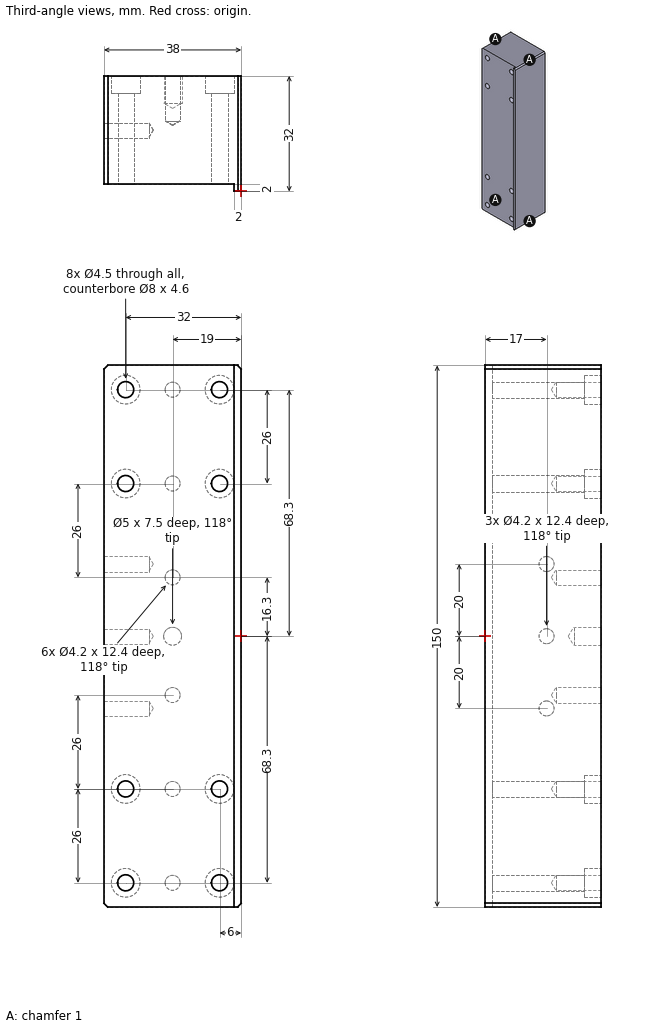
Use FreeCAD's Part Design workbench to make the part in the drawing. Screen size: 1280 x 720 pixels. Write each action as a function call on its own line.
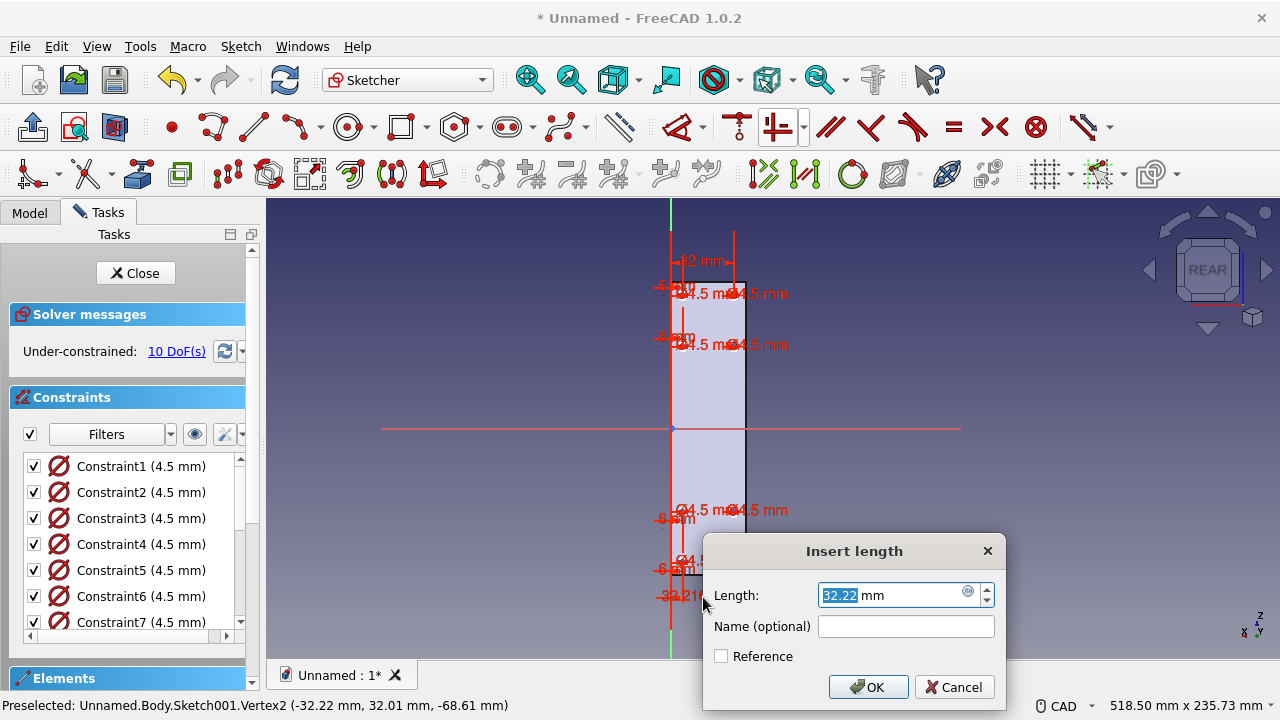
text(32)
key(Return)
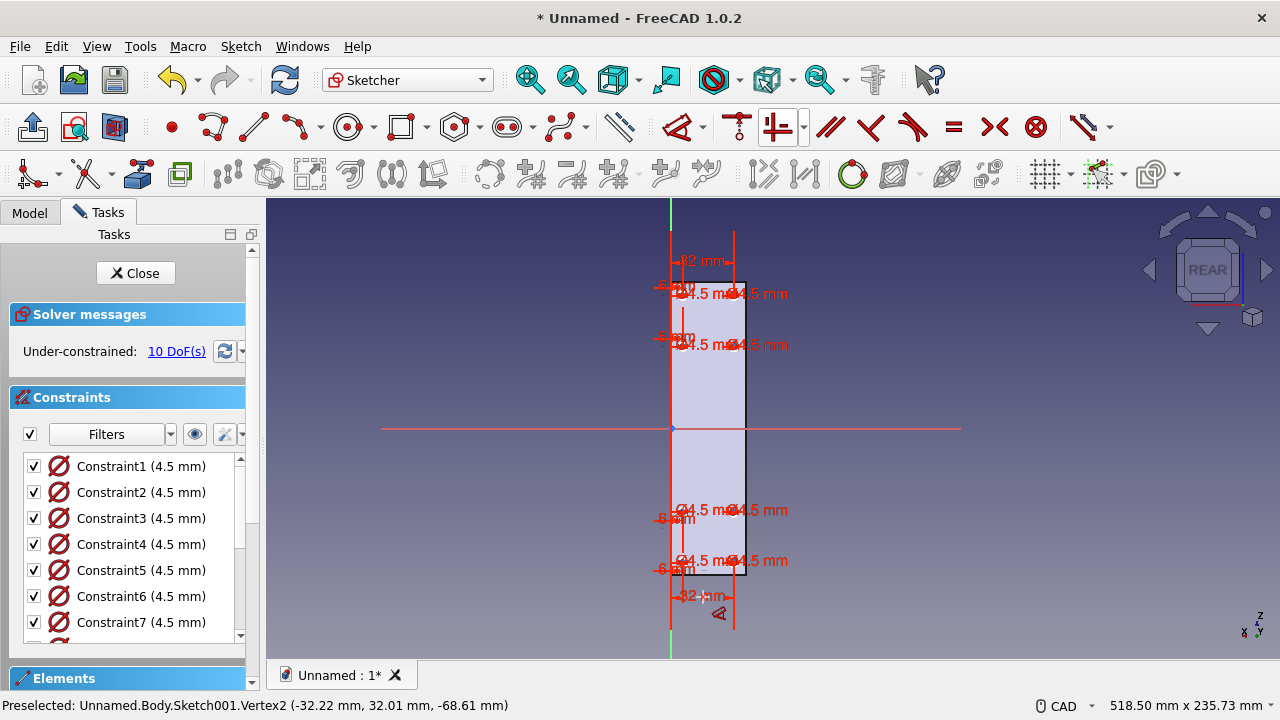
click(734, 512)
click(702, 546)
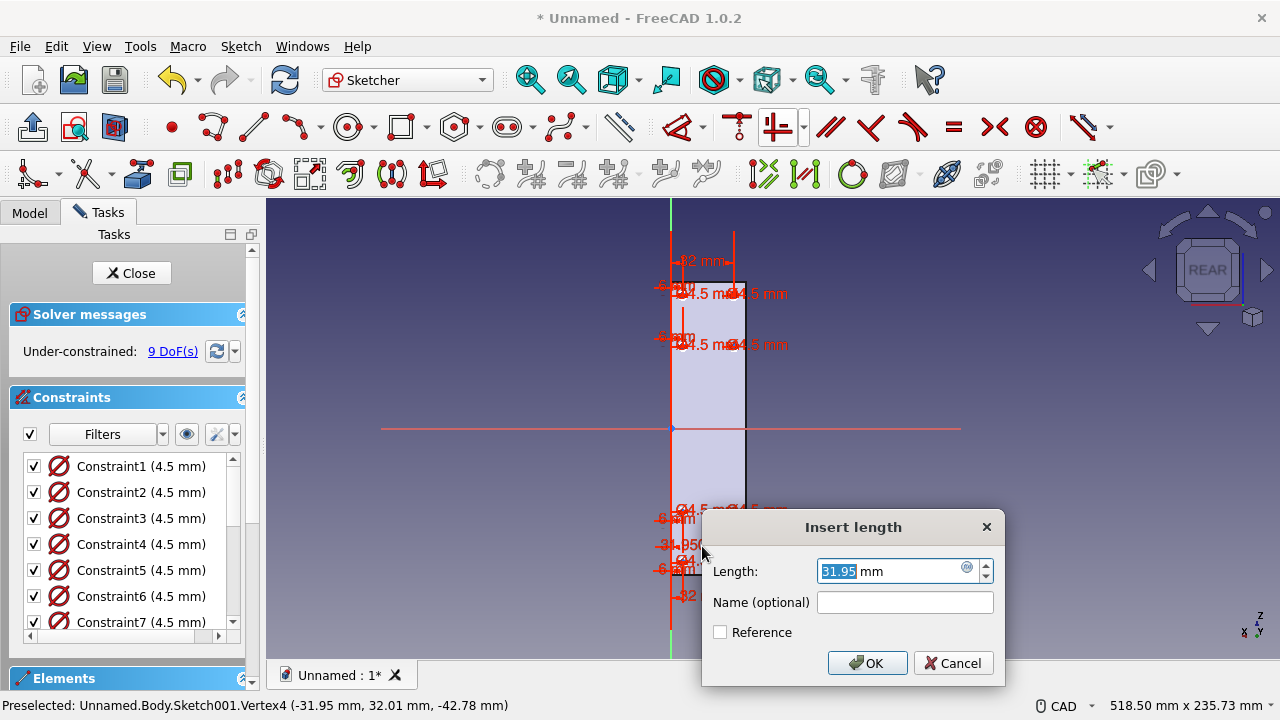
text(32)
key(Return)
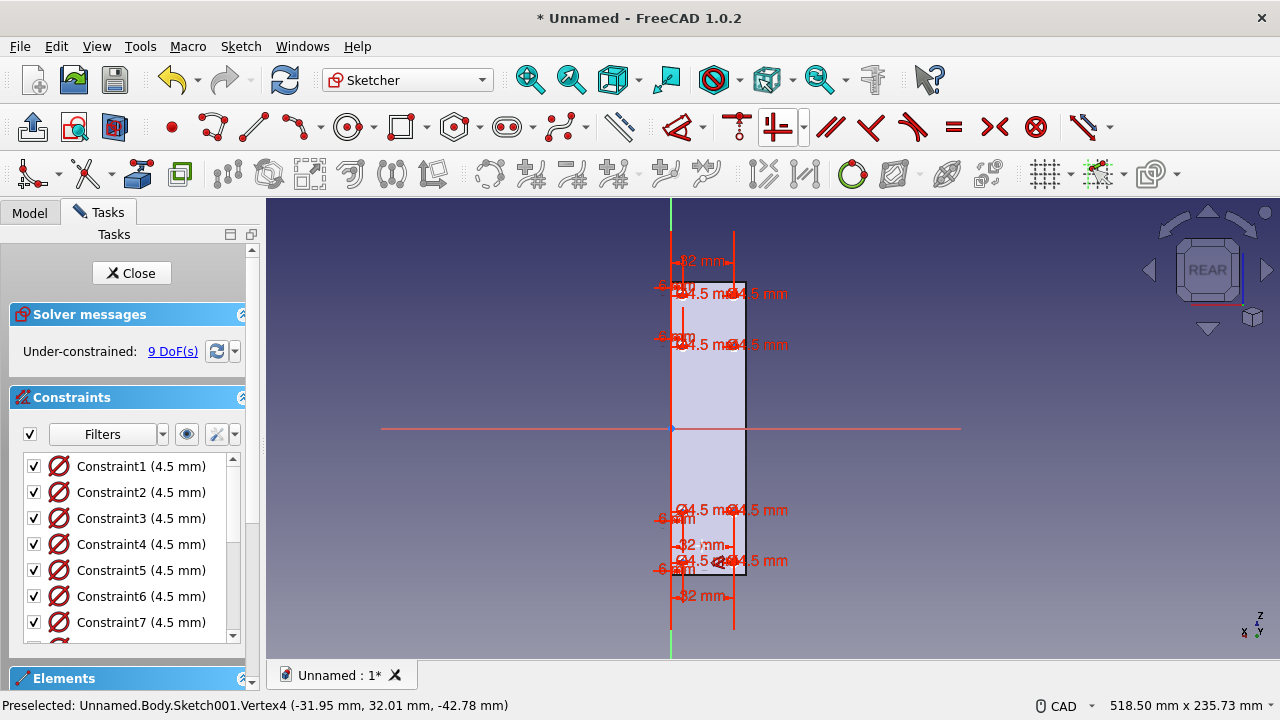
click(734, 347)
click(703, 313)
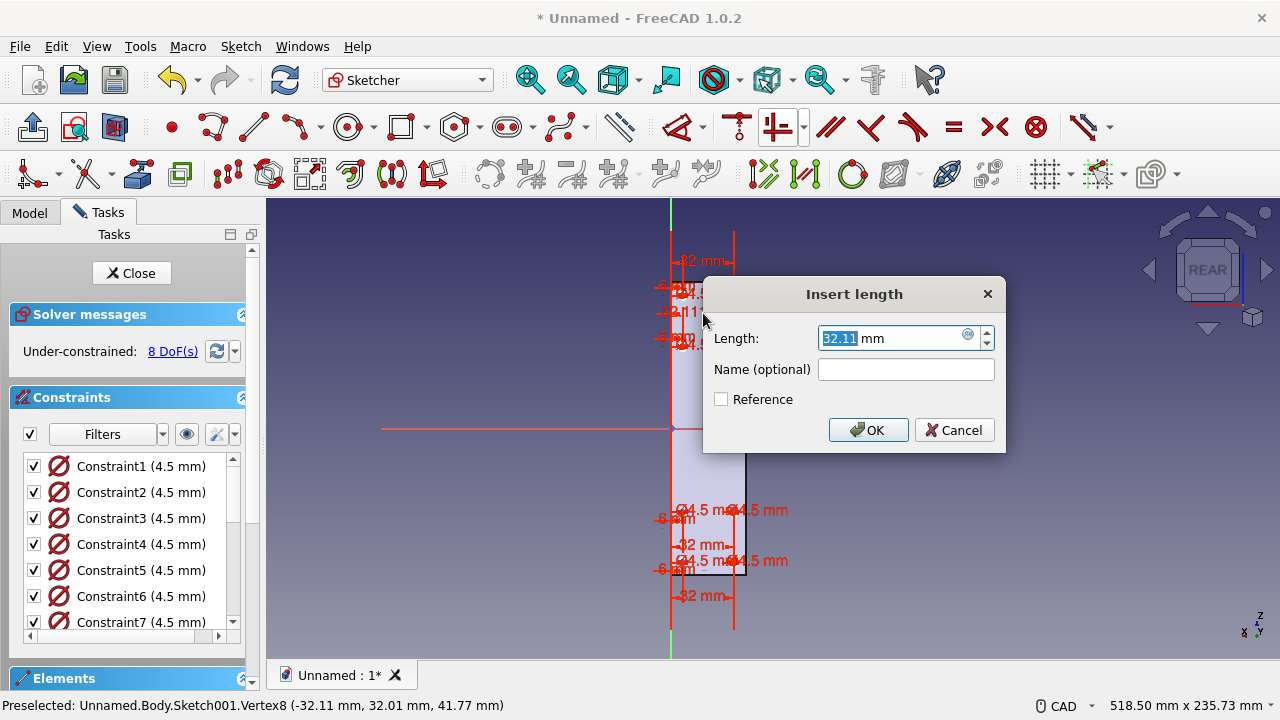
text(32)
key(Return)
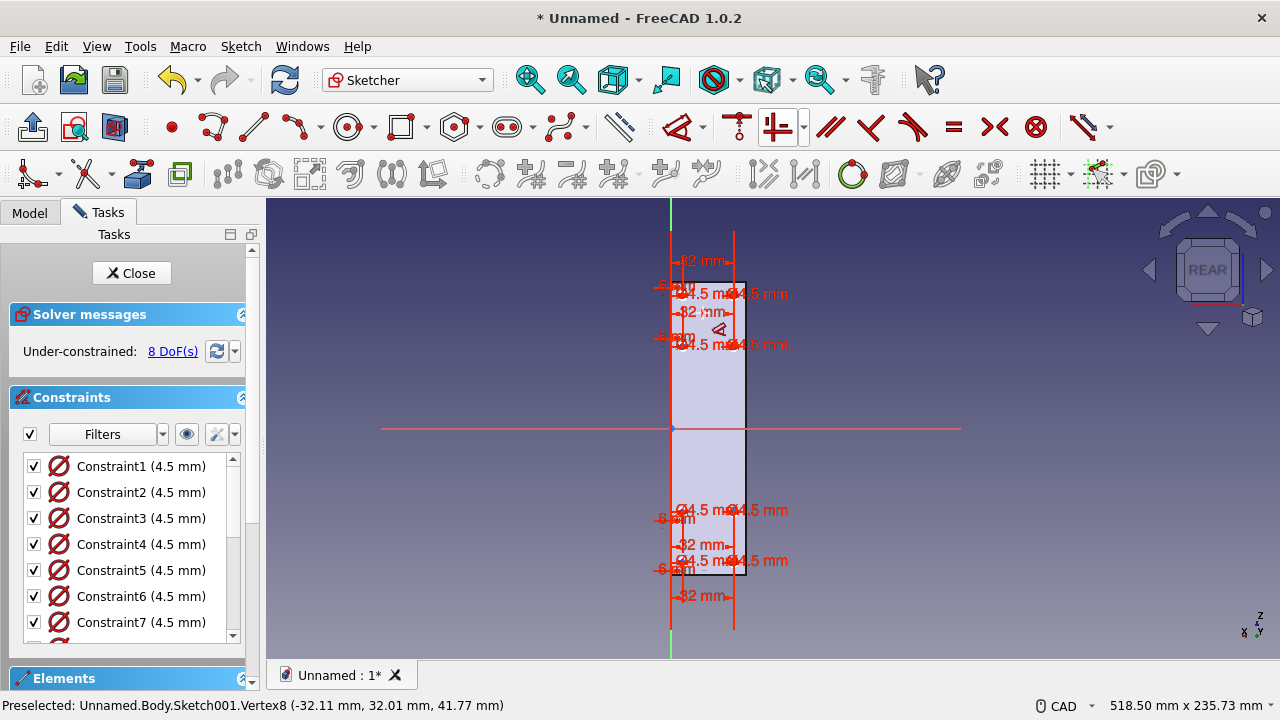
click(734, 563)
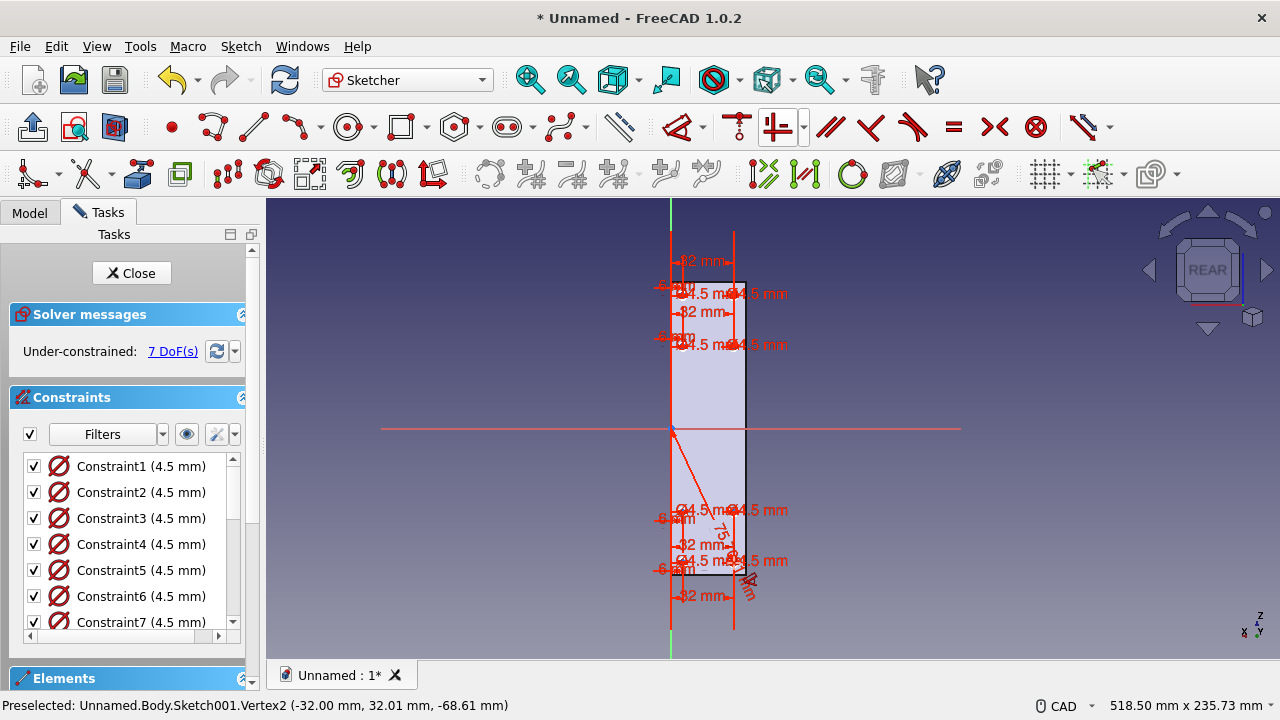
click(683, 512)
click(768, 526)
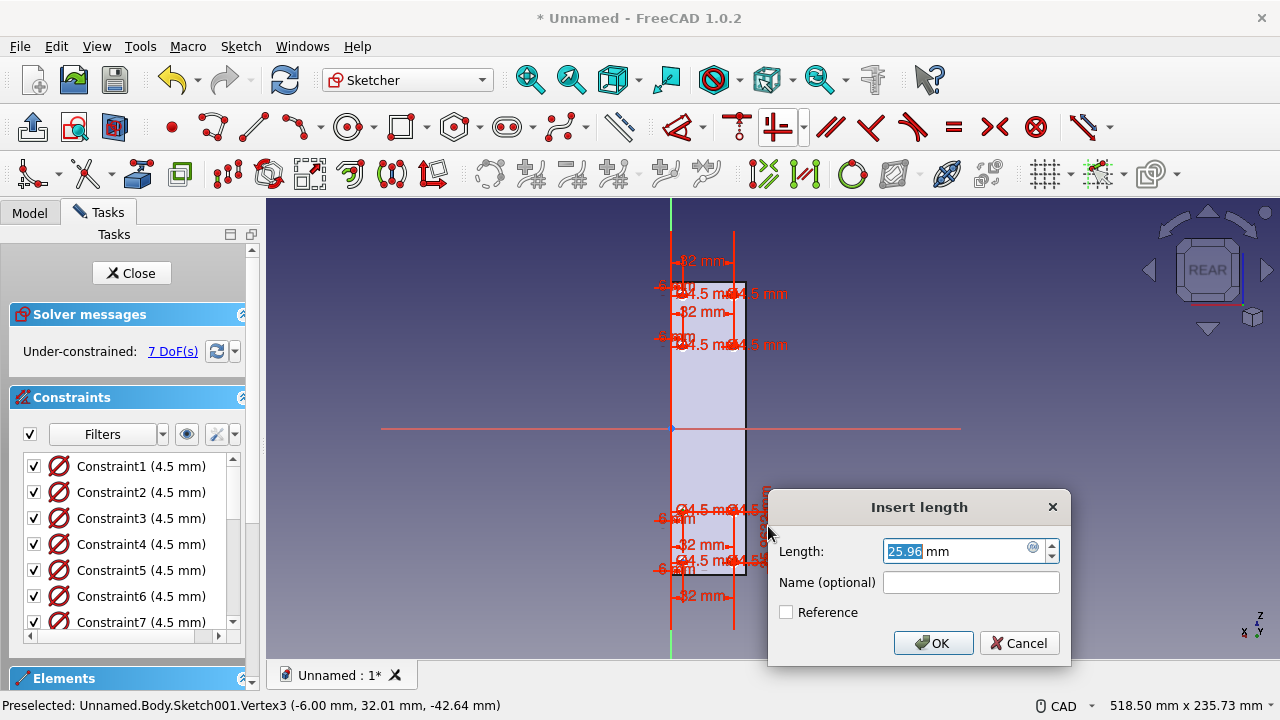
text(26)
key(Return)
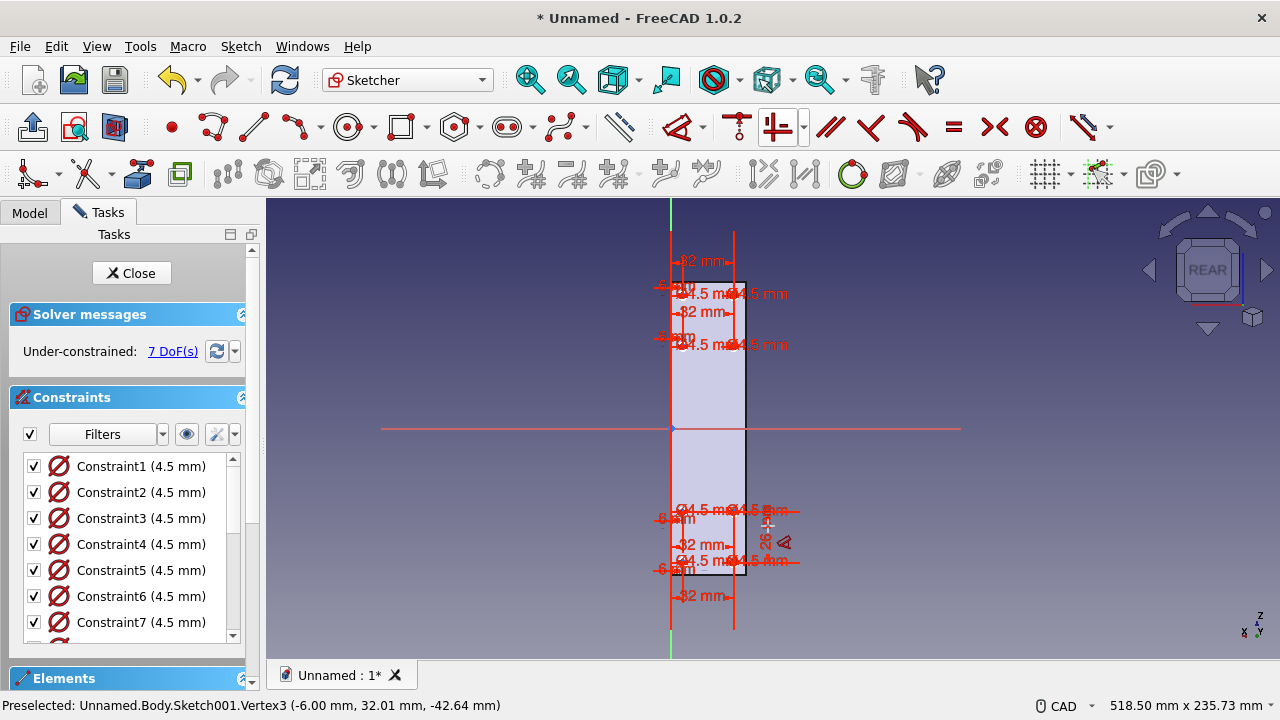
click(734, 563)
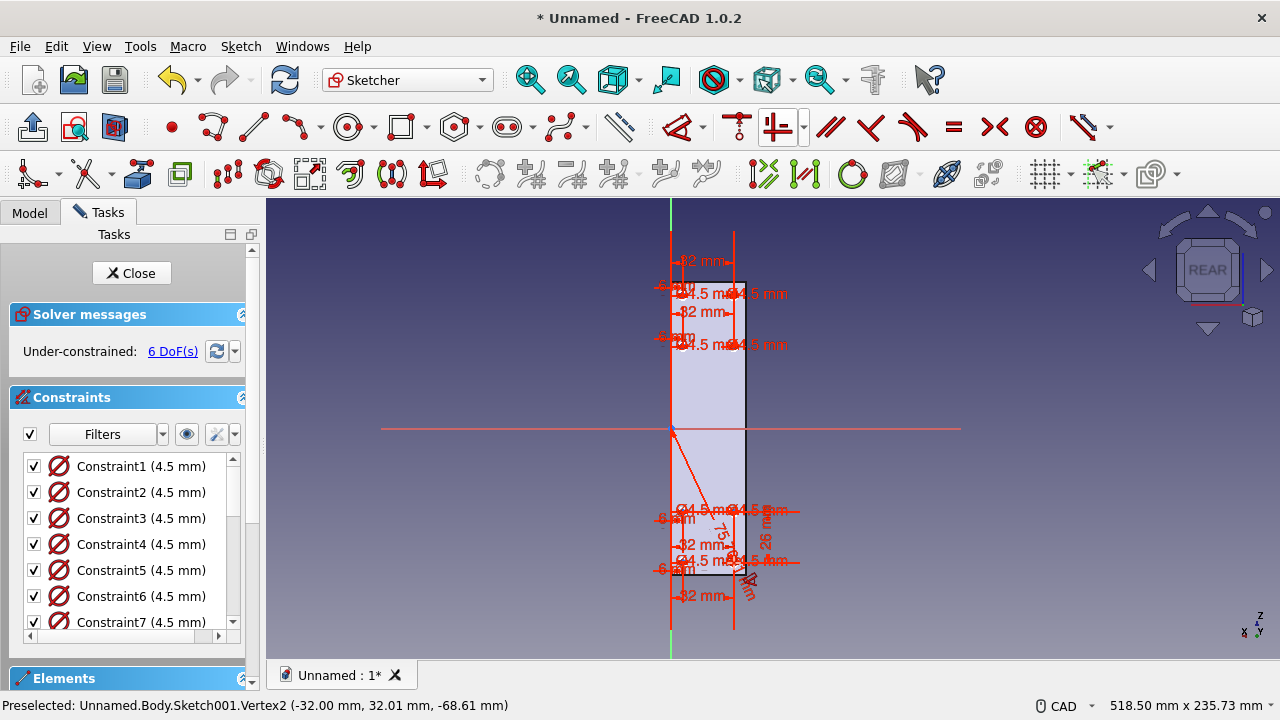
click(734, 512)
click(792, 549)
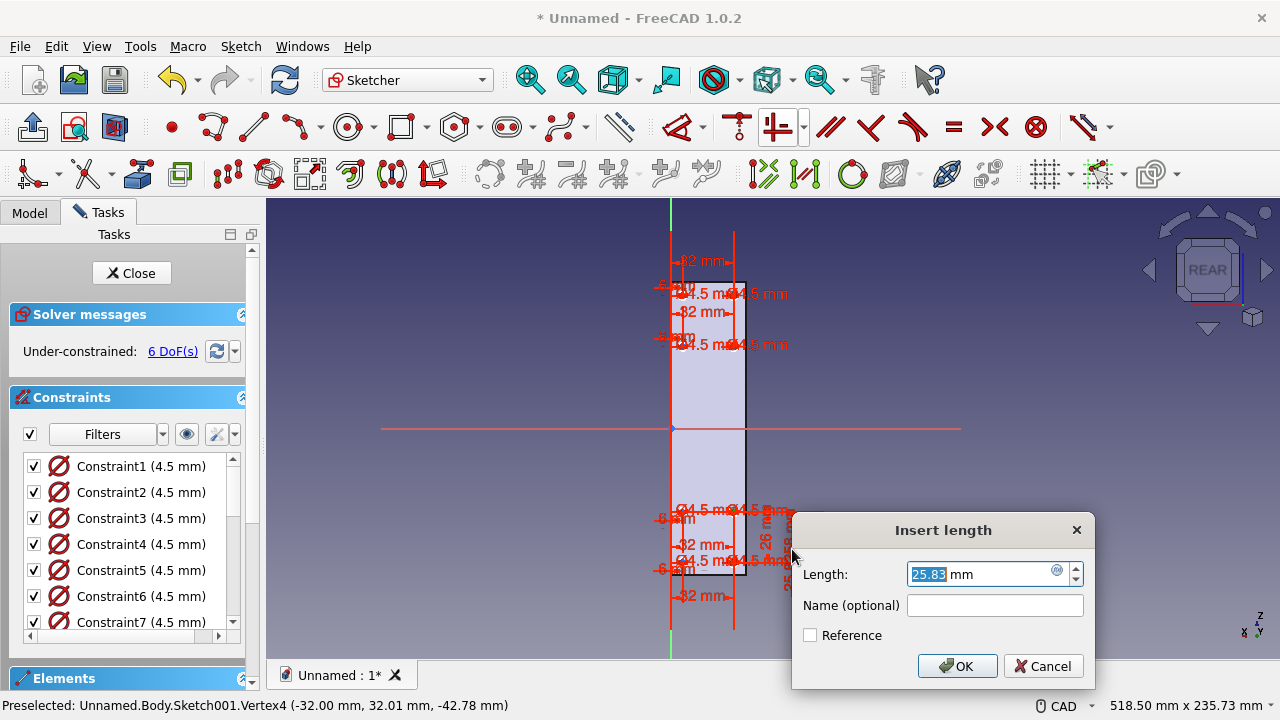
text(26)
key(Return)